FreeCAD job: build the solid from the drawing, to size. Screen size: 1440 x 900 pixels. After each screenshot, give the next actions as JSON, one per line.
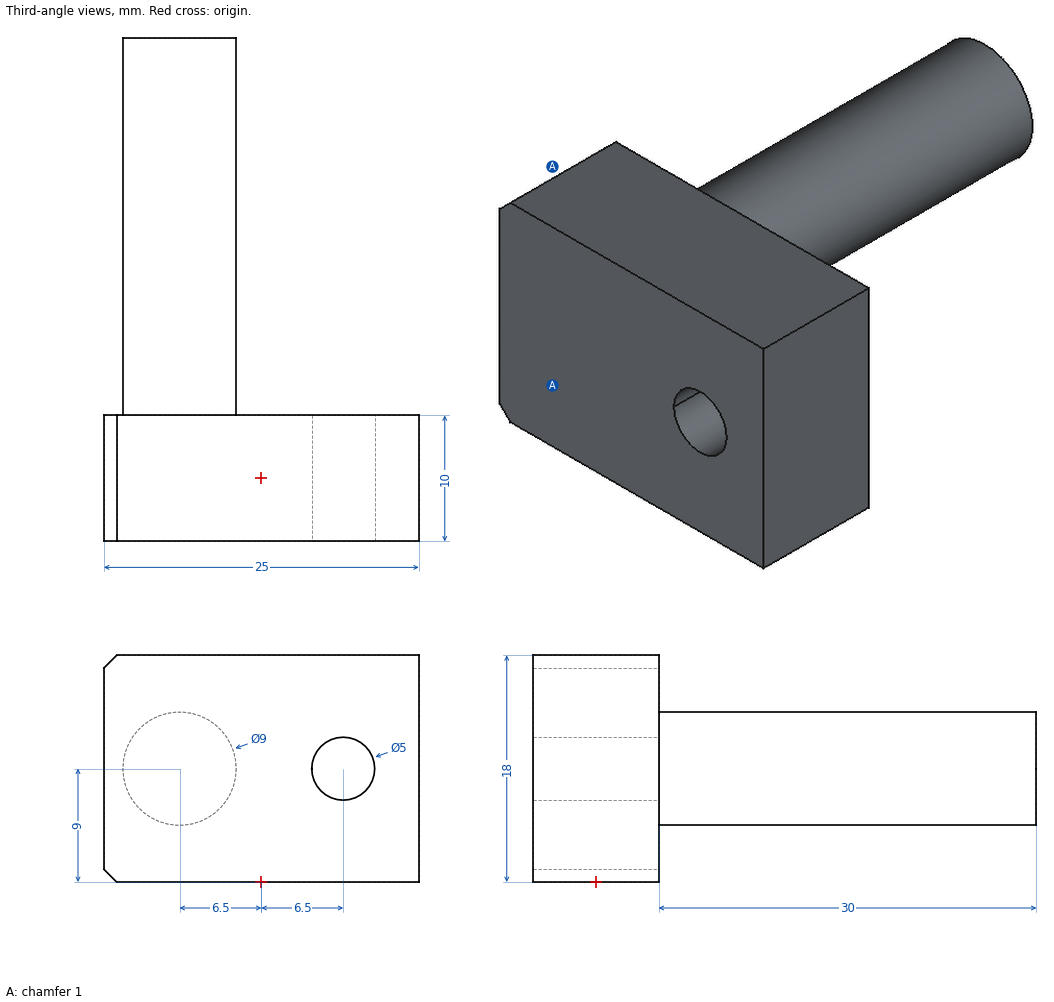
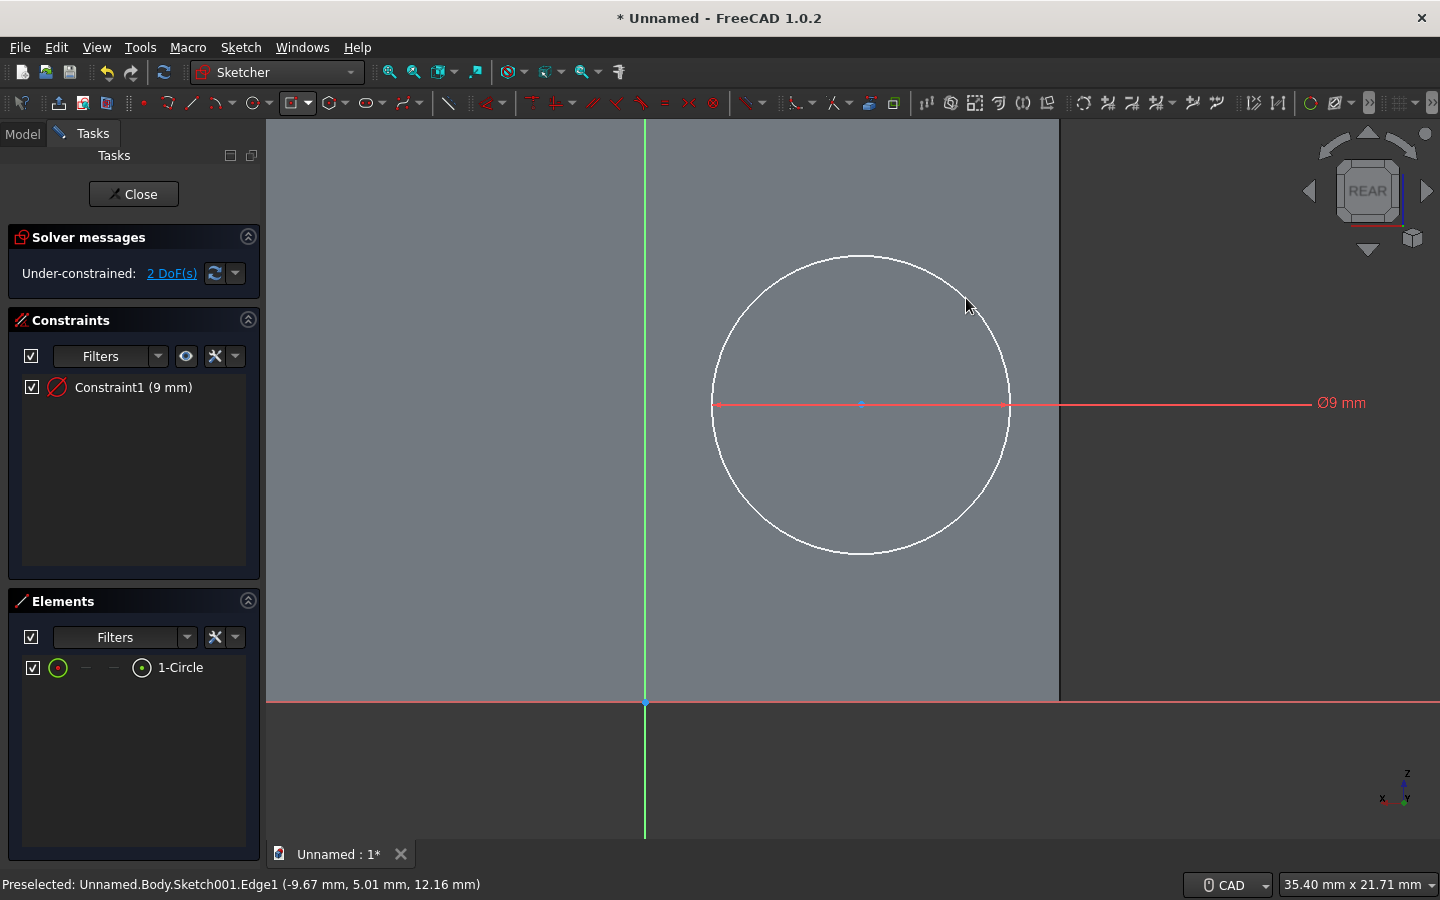
{"action": "left_click", "coordinate": [861, 405]}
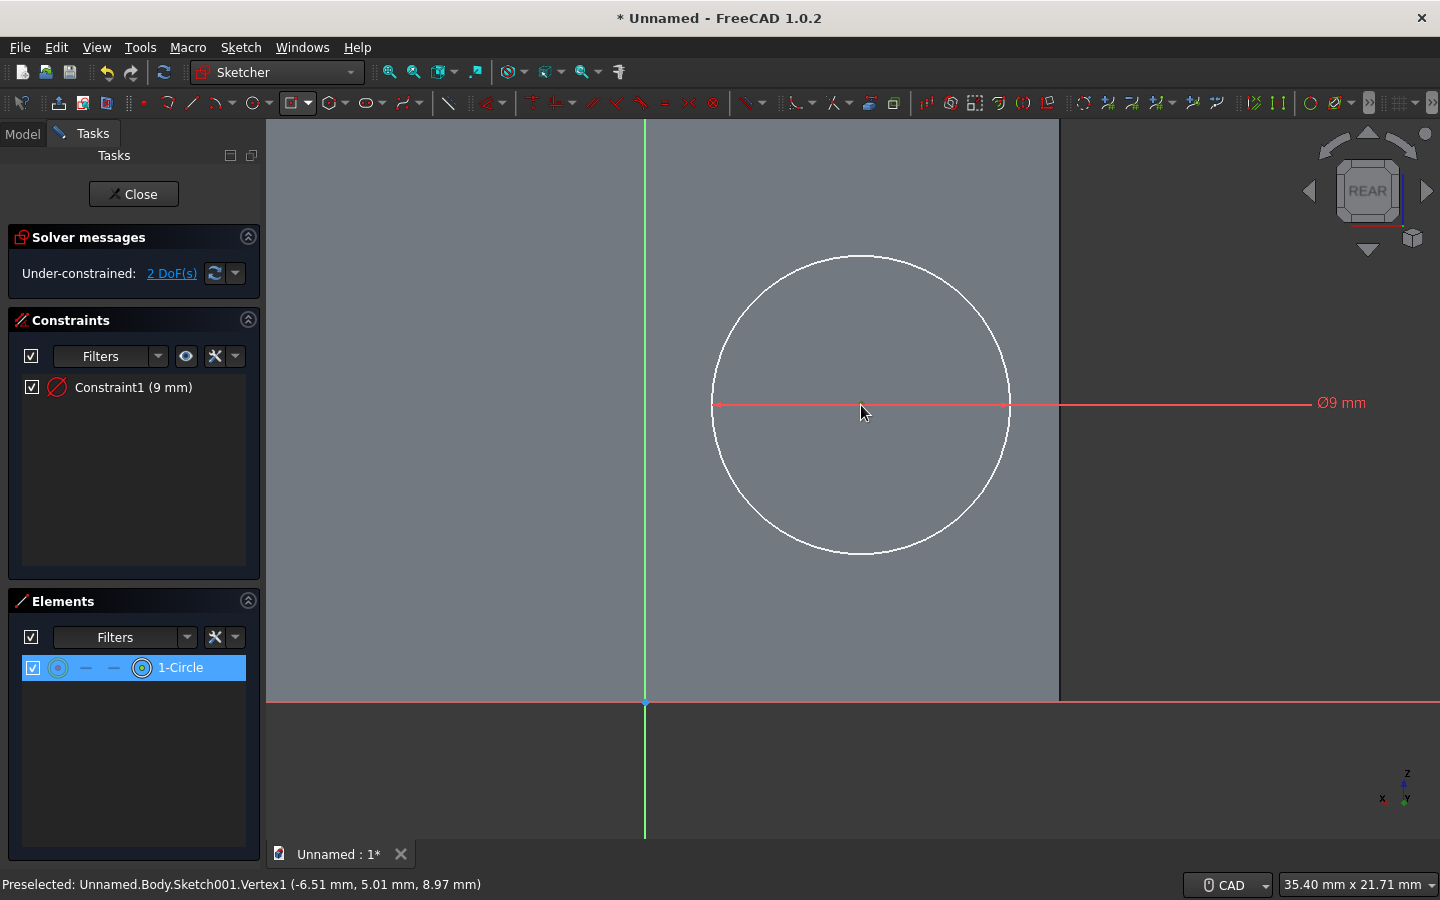
{"action": "key", "text": "i"}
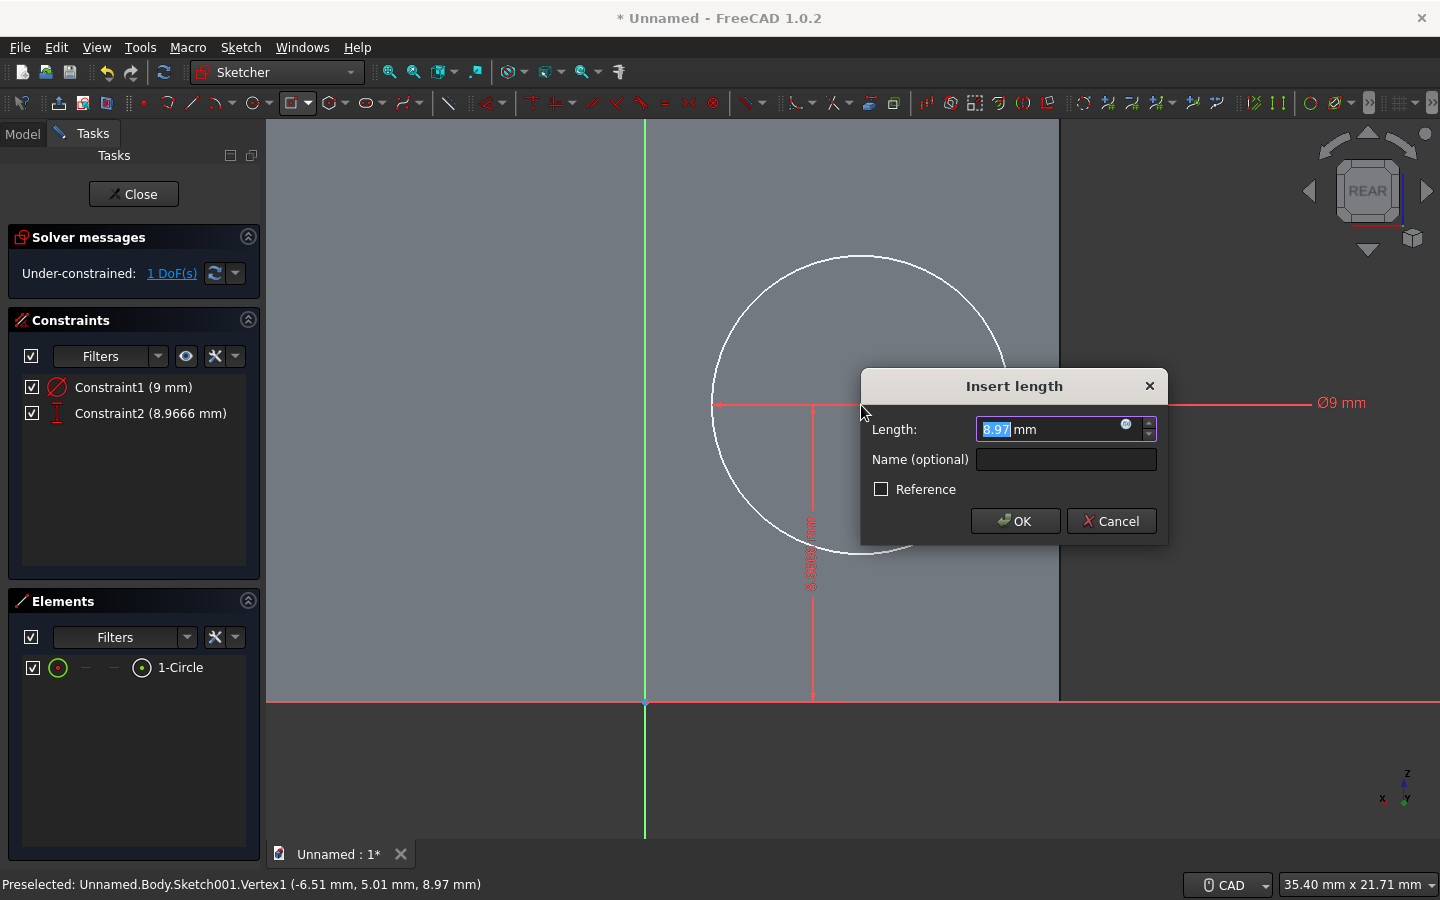
{"action": "type", "text": "9"}
{"action": "key", "text": "Return"}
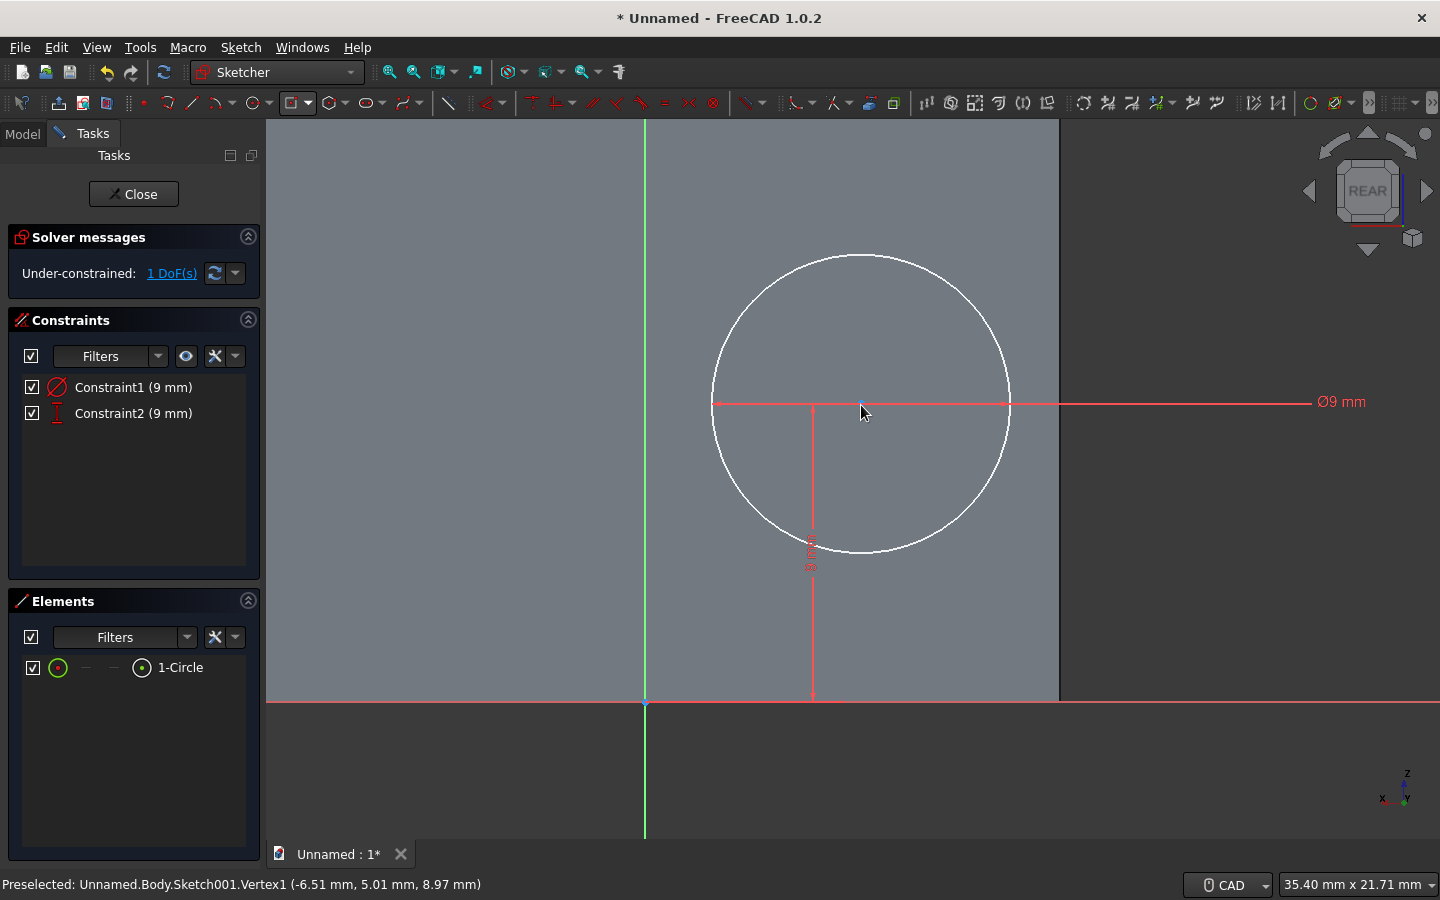
{"action": "left_click", "coordinate": [861, 404]}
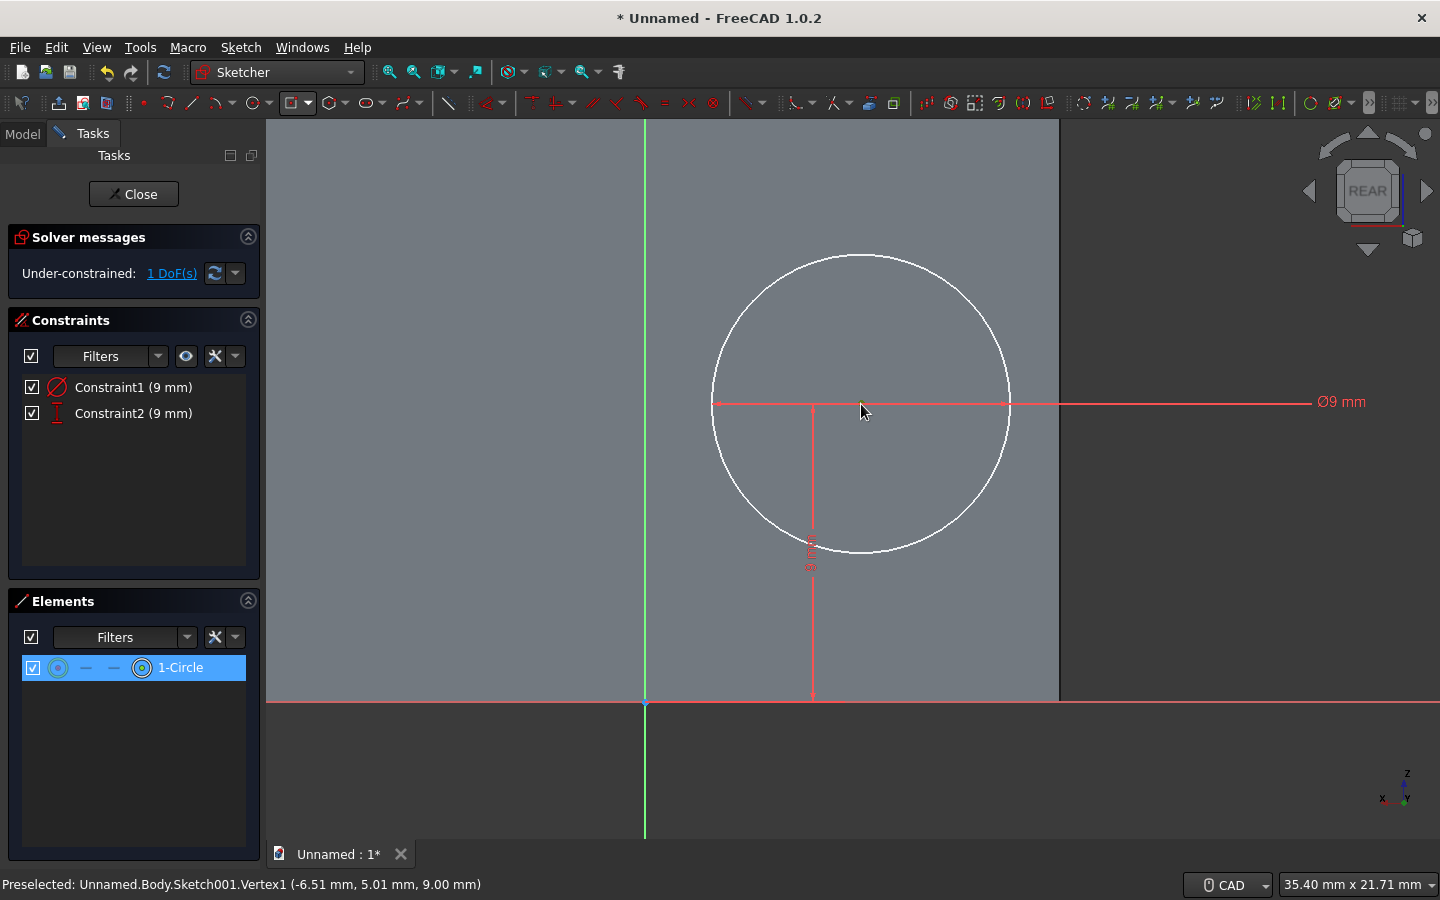
{"action": "key", "text": "l"}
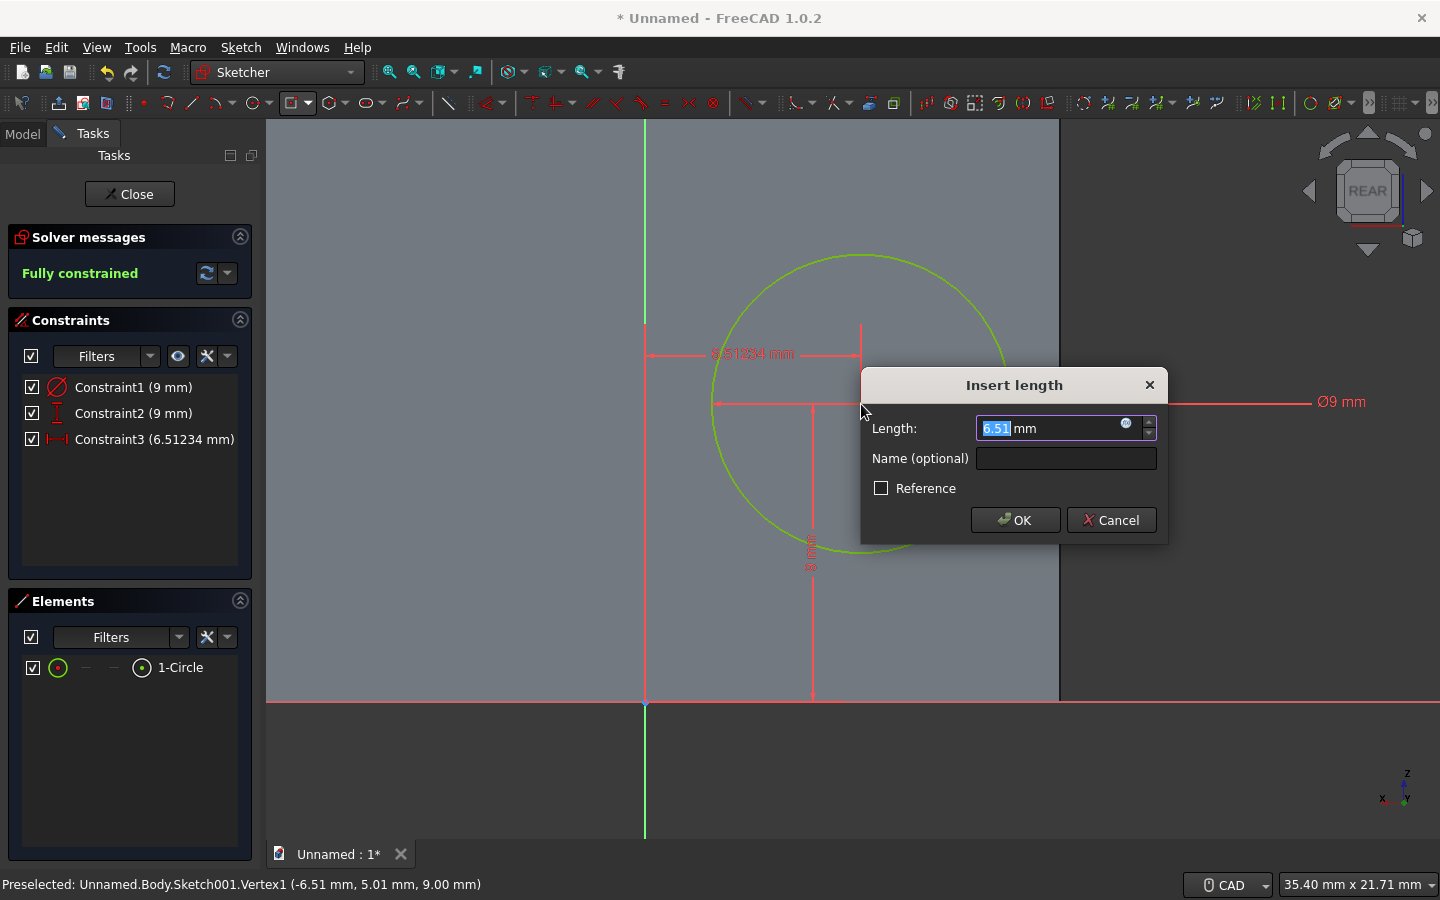
{"action": "type", "text": "6.5"}
{"action": "key", "text": "Return"}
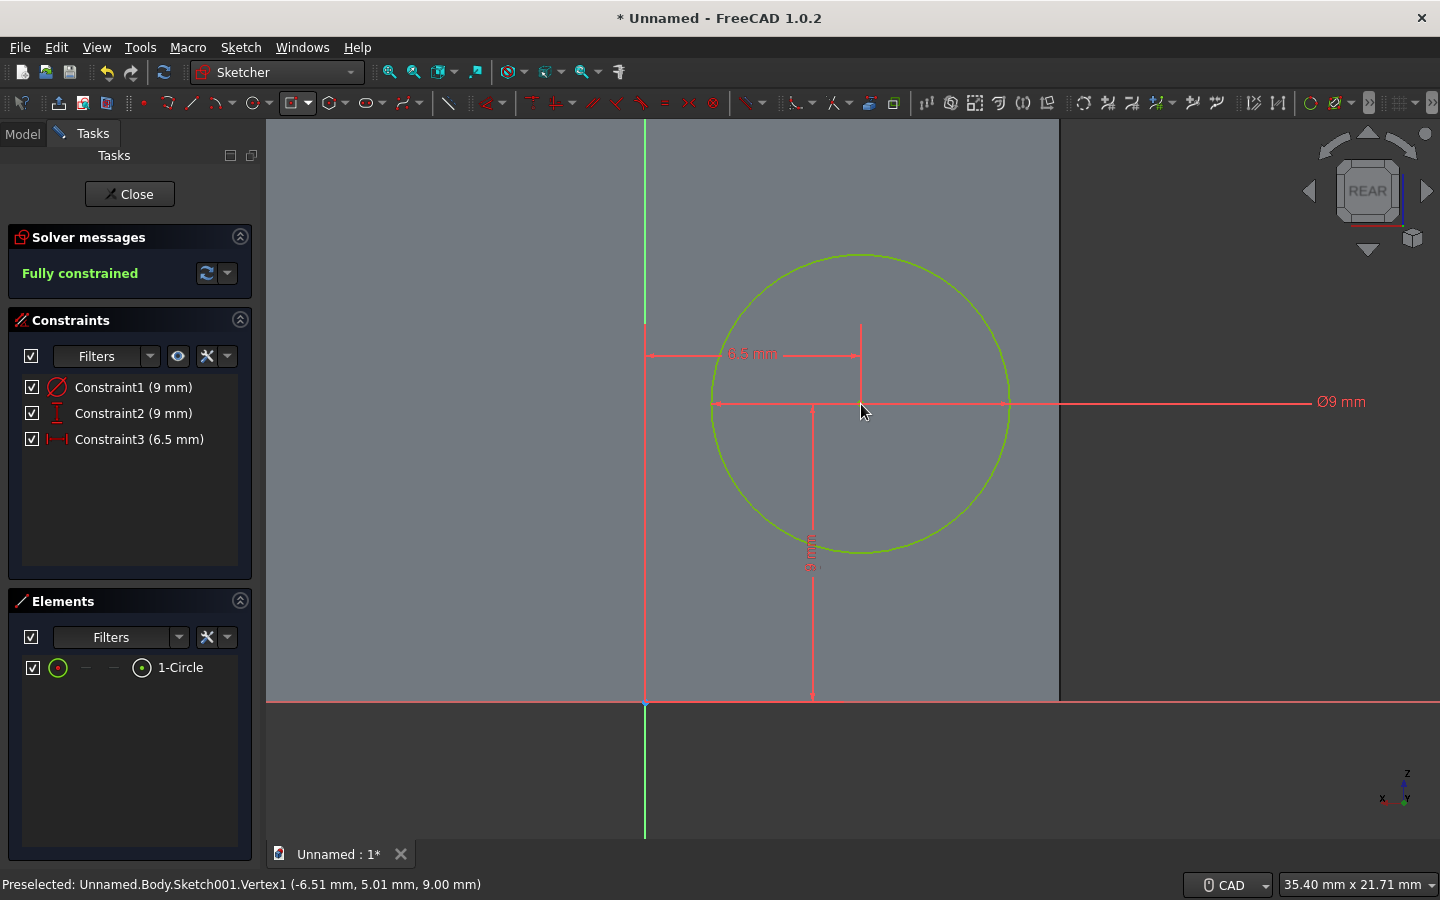
{"action": "left_click", "coordinate": [130, 194]}